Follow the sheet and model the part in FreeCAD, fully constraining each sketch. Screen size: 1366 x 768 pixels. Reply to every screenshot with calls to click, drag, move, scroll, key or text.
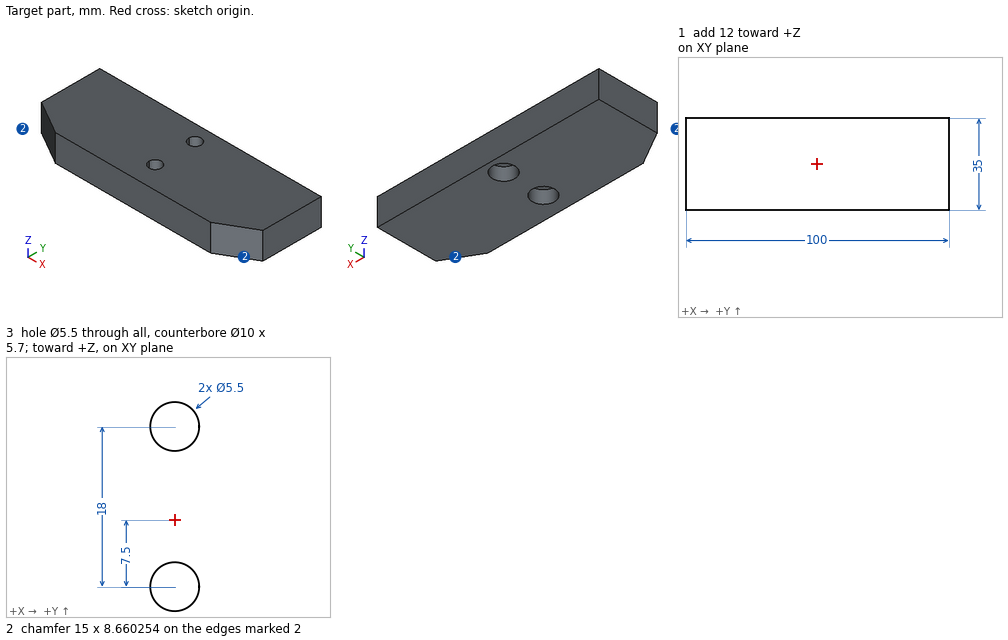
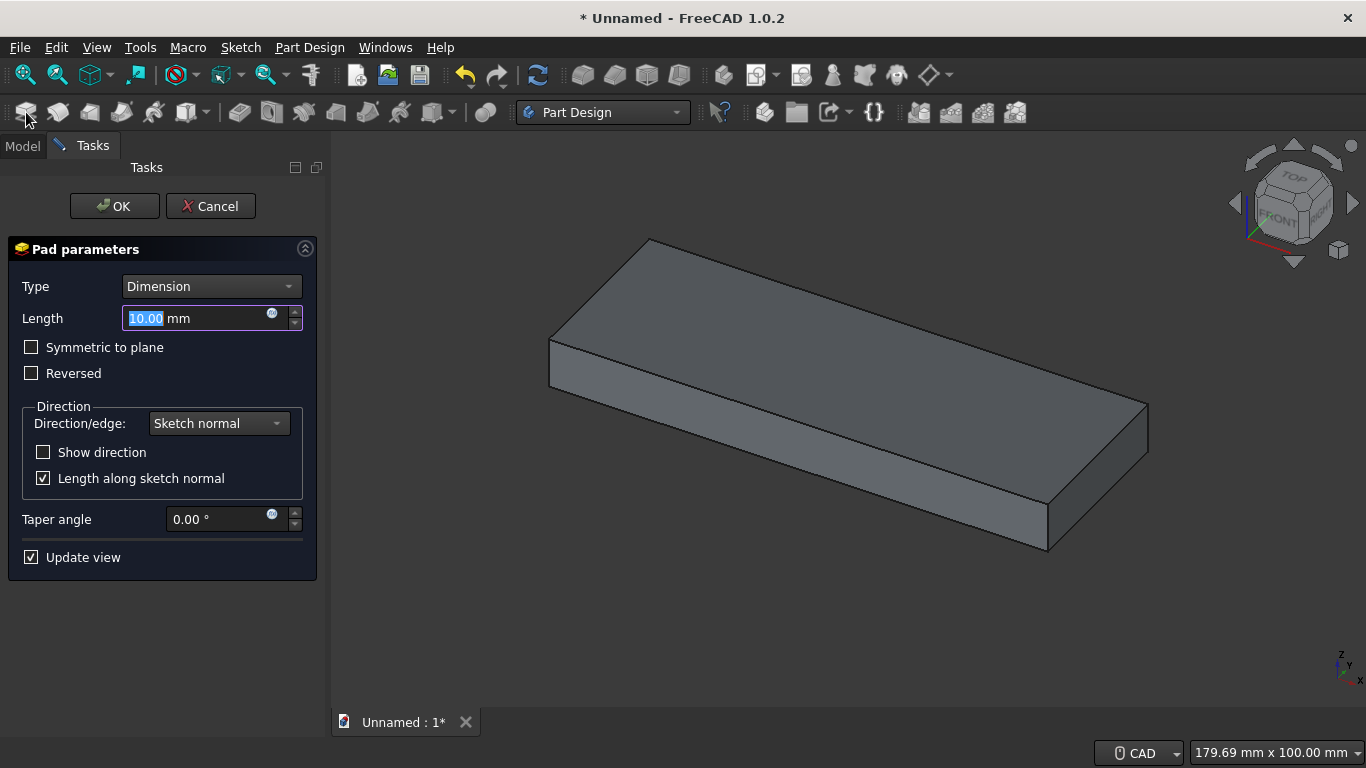
text(12)
key(Tab)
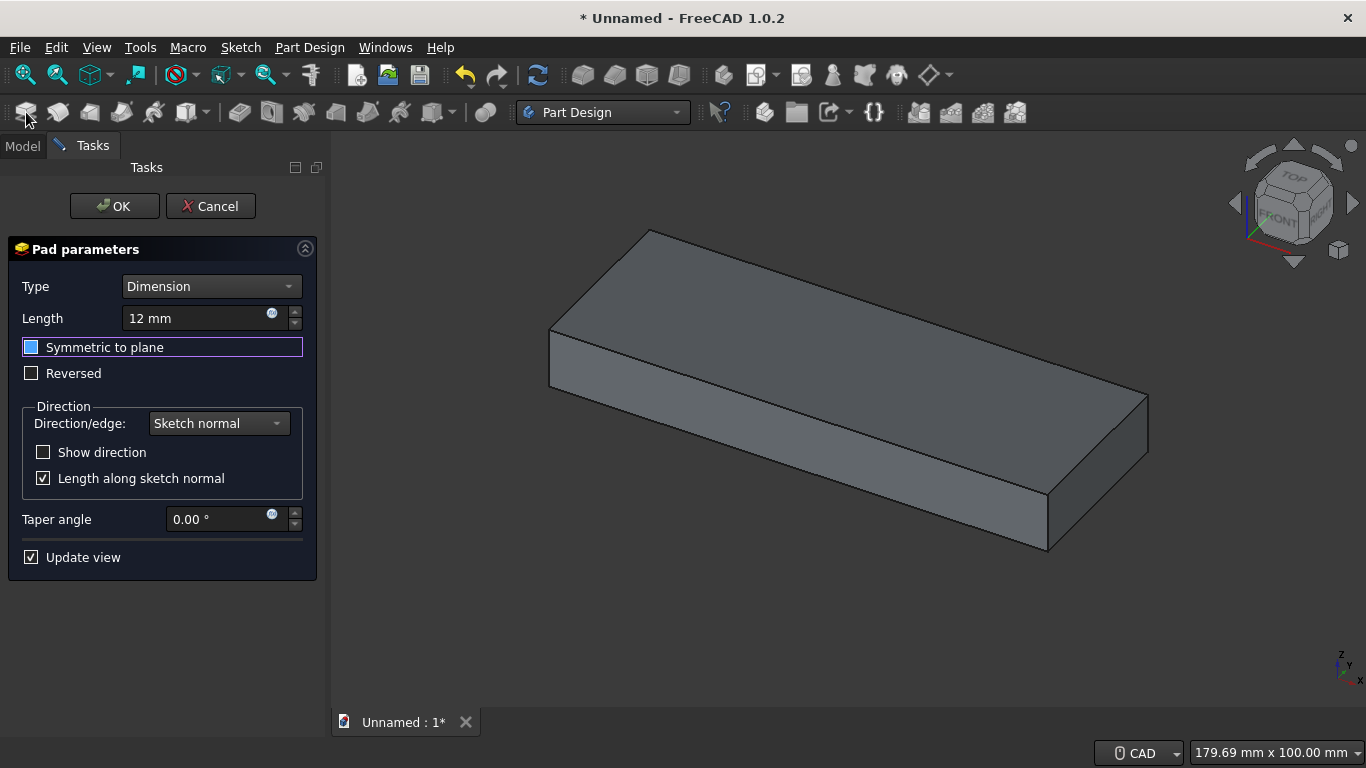
click(115, 206)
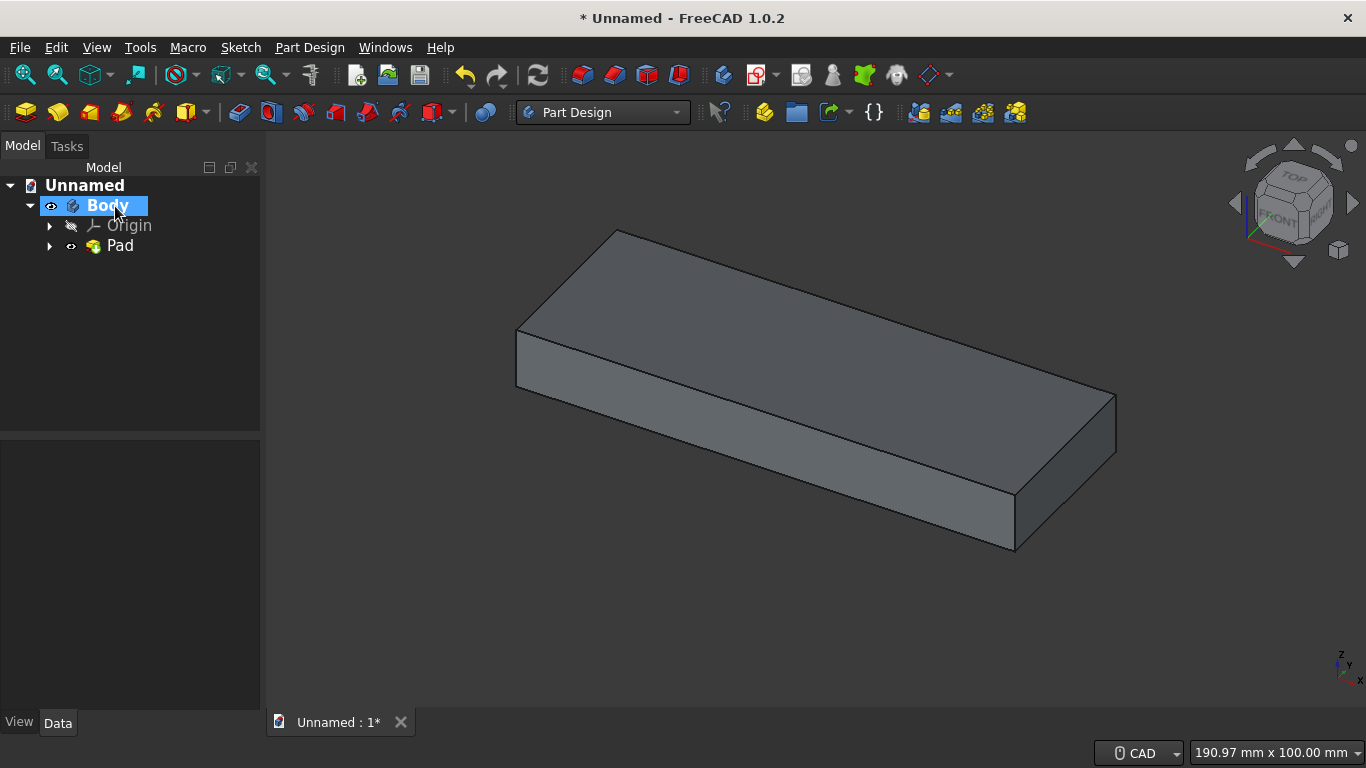
click(1015, 522)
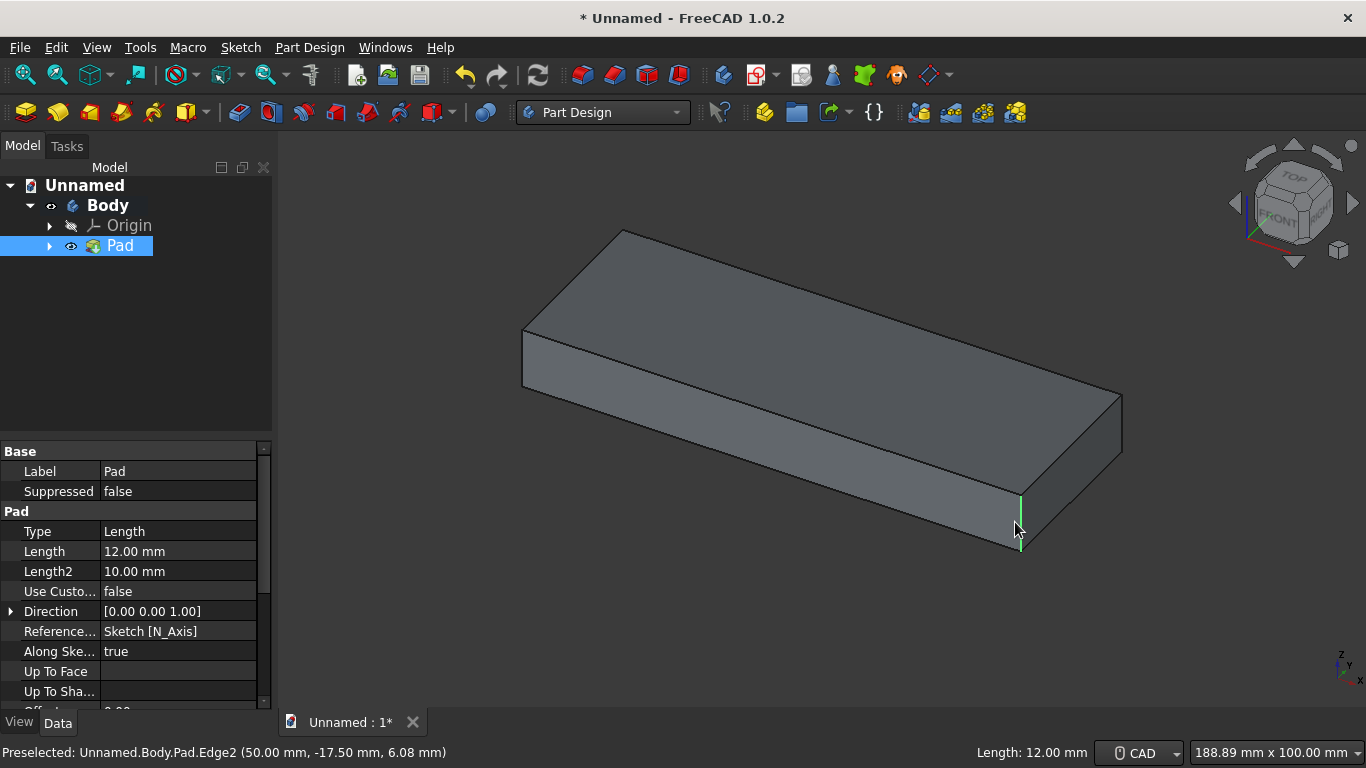
key(0)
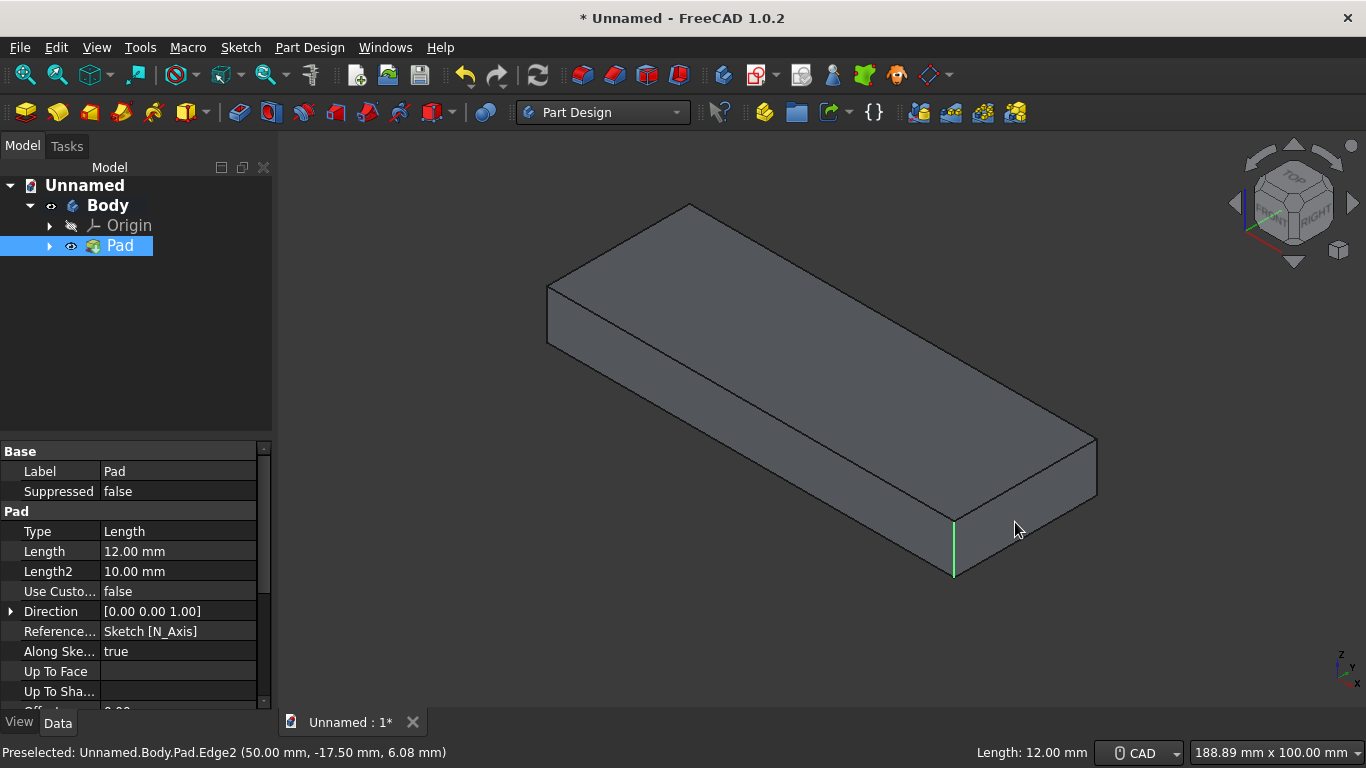
key(2)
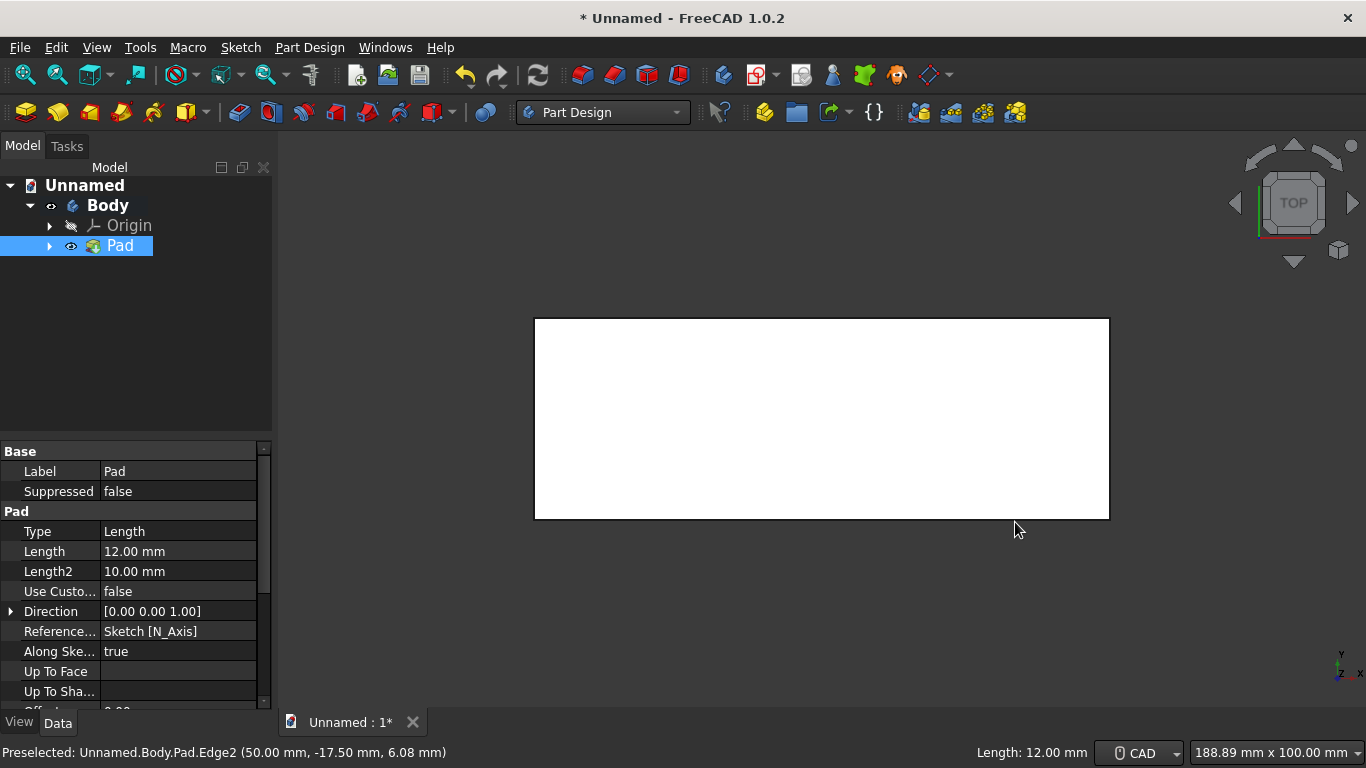
key(1)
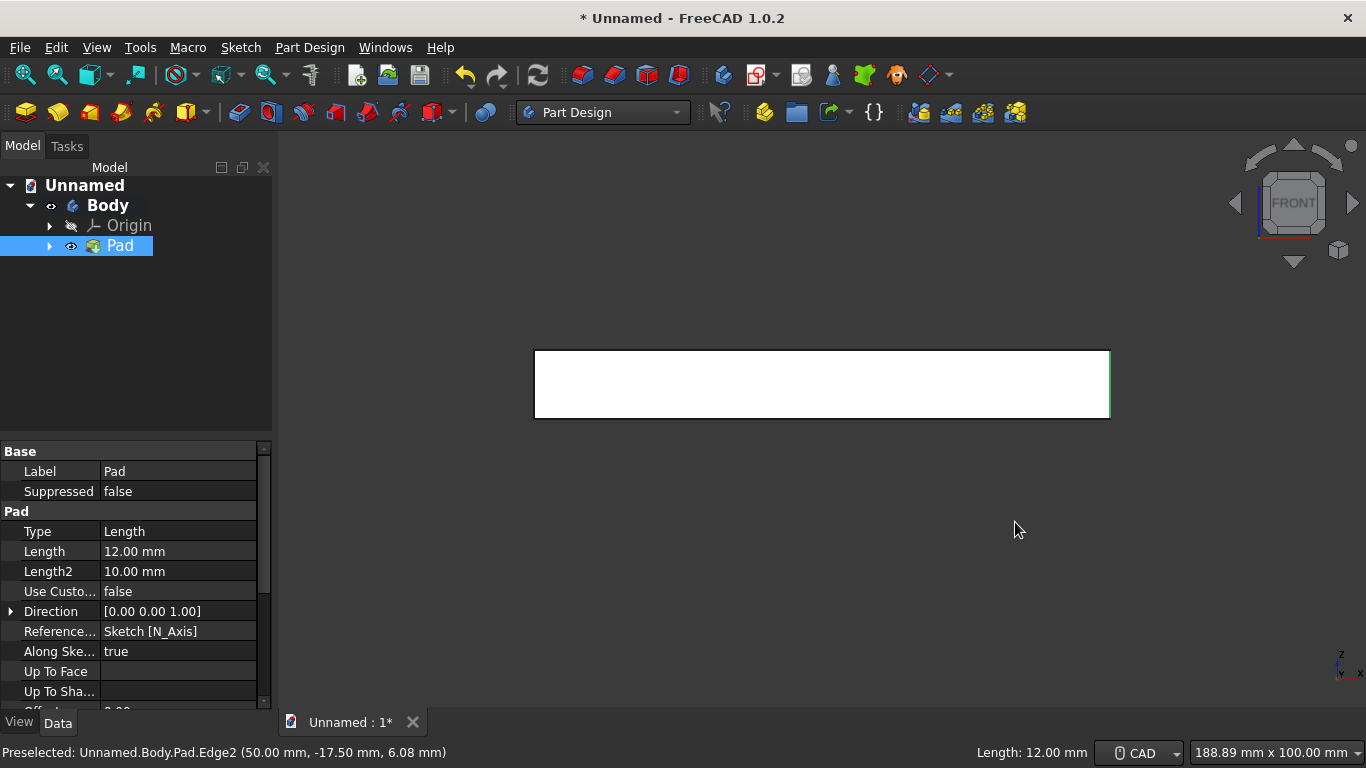
click(534, 383, ctrl)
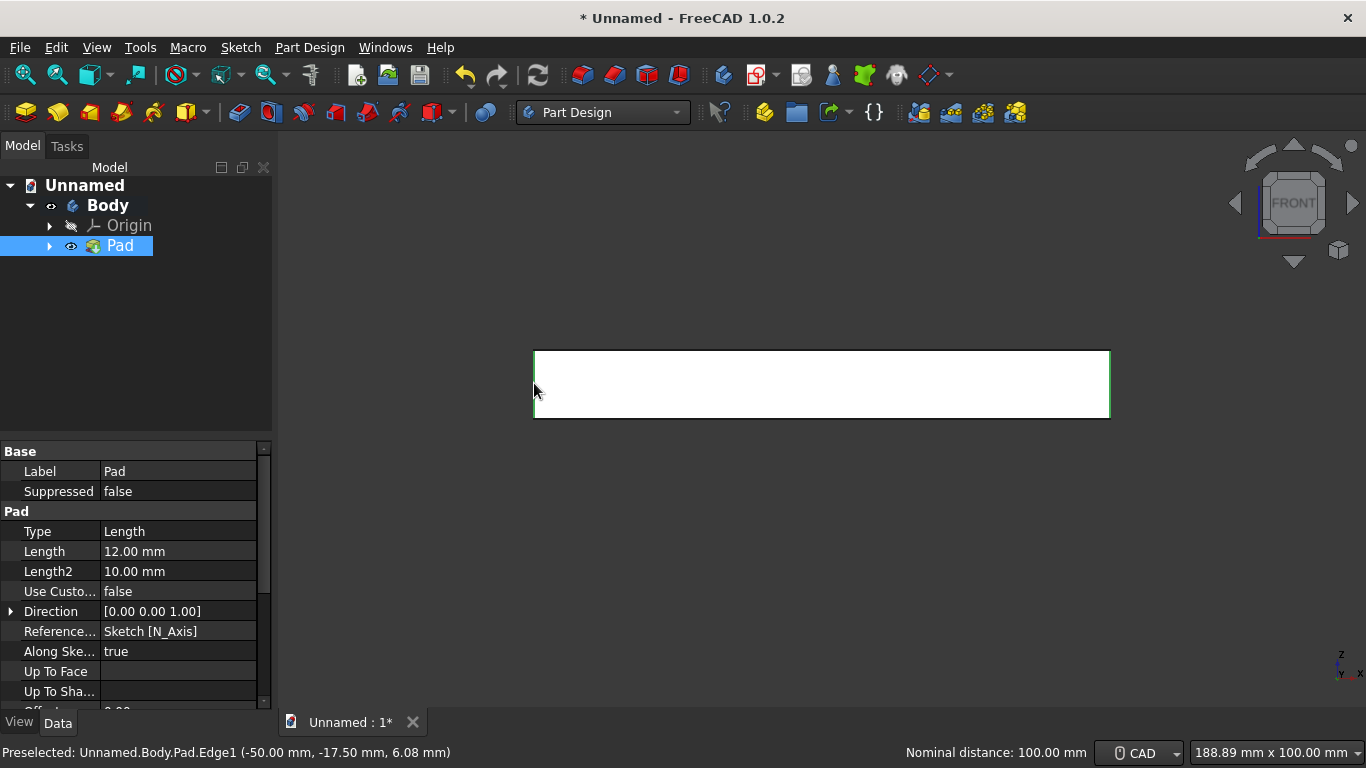
click(616, 76)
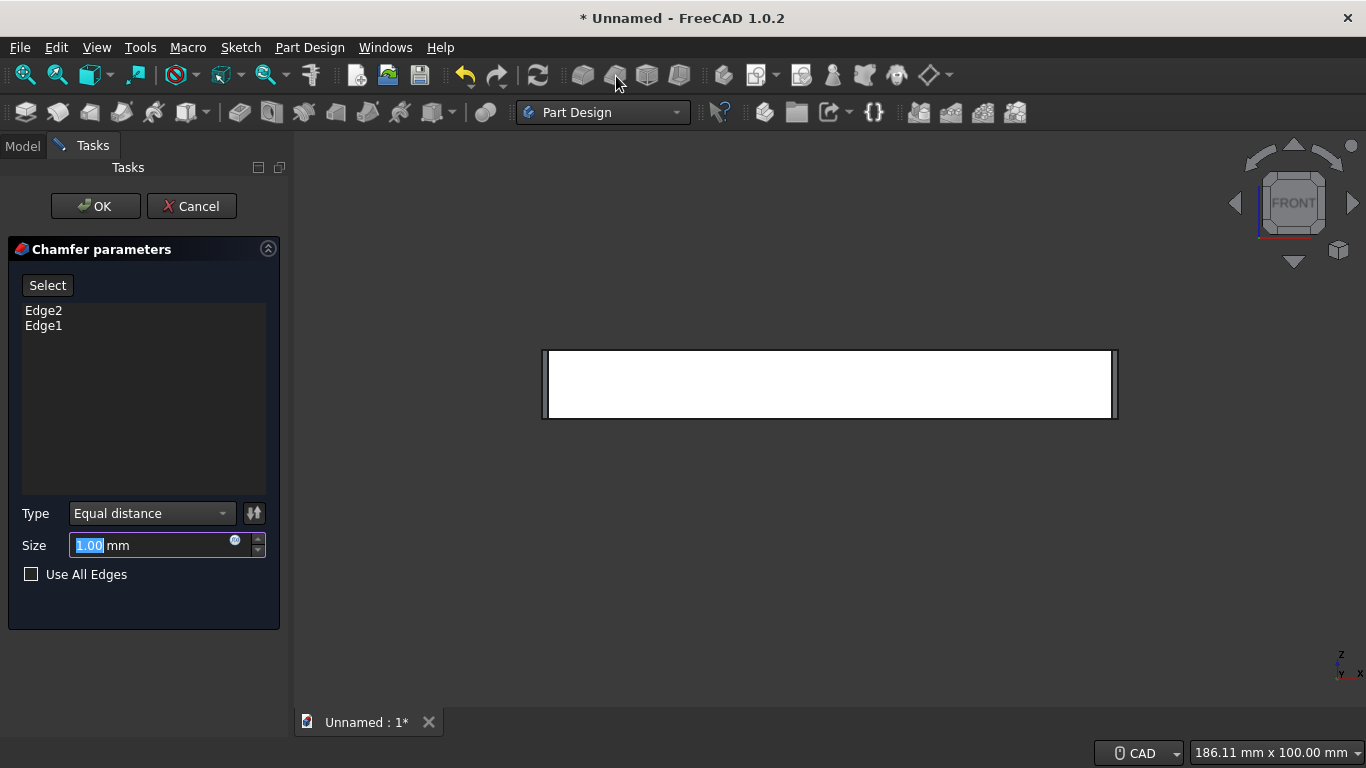
text(15)
key(Tab)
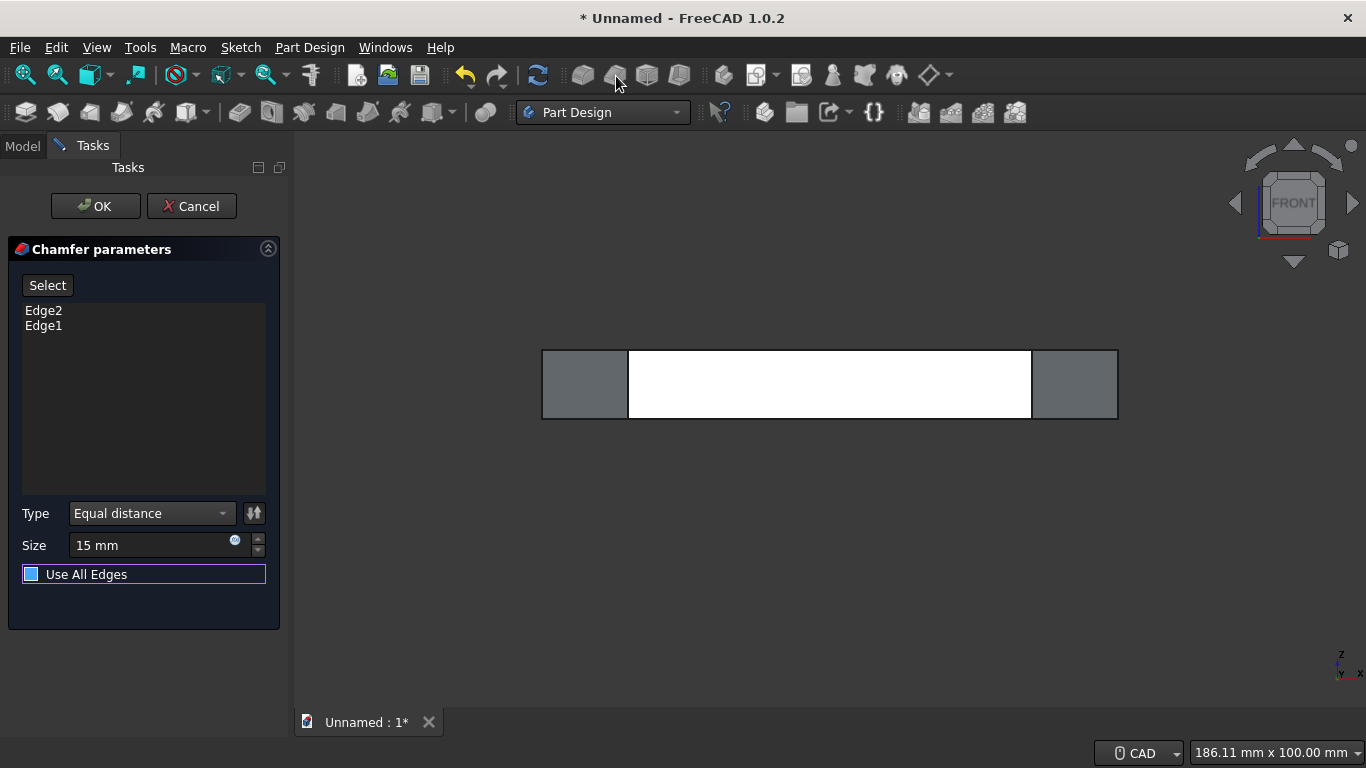
click(153, 514)